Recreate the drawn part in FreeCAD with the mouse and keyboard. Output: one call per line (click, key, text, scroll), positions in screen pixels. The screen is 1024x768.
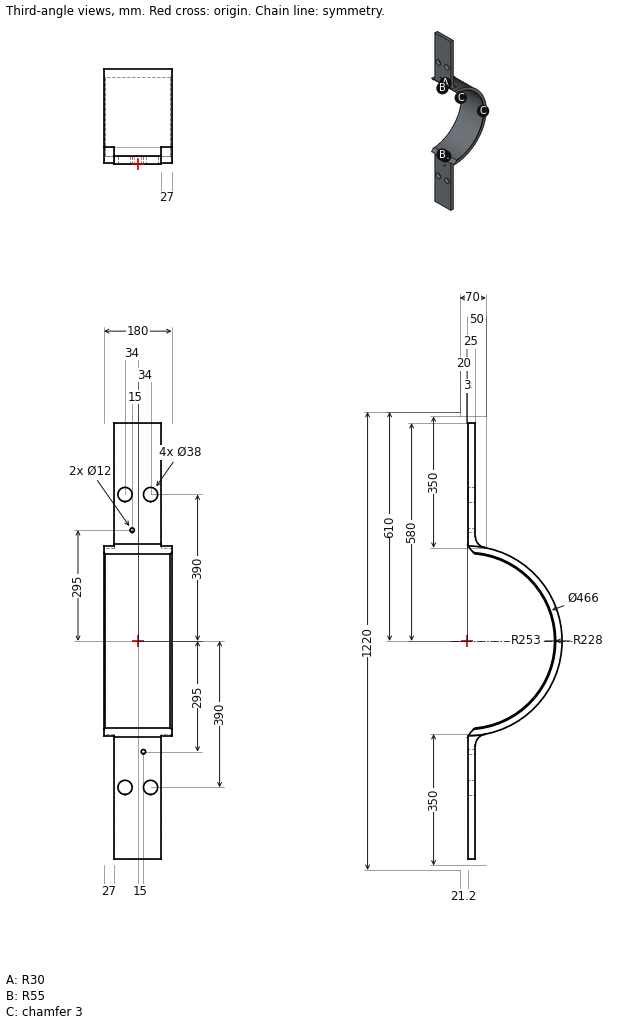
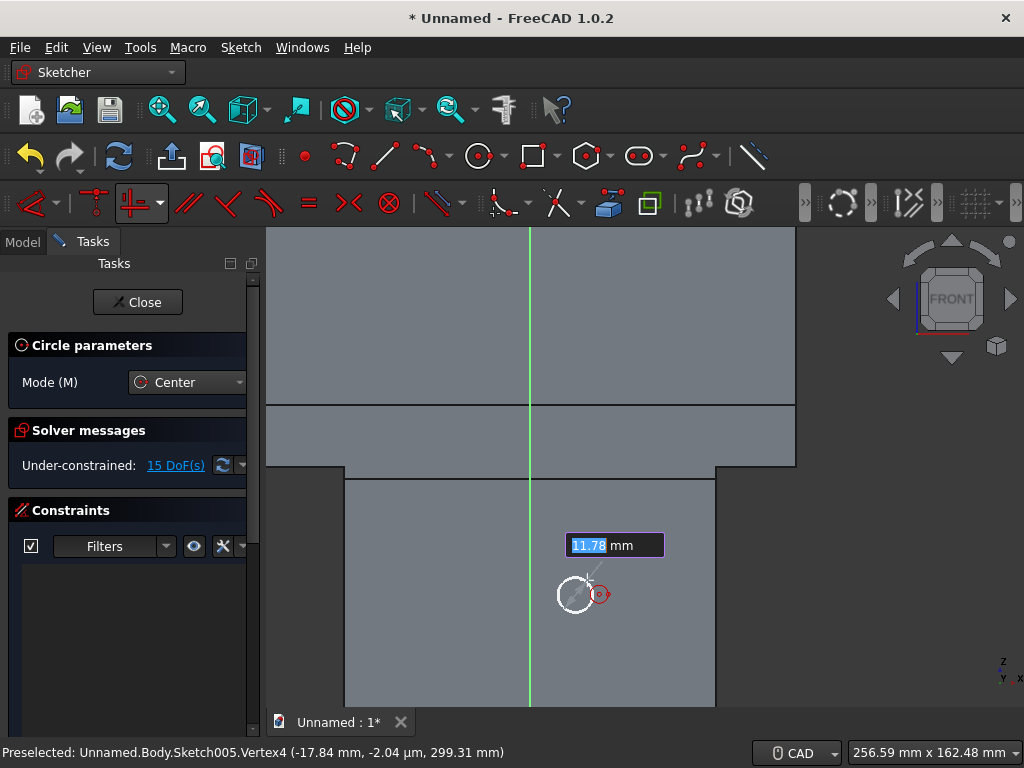
click(587, 579)
key(Escape)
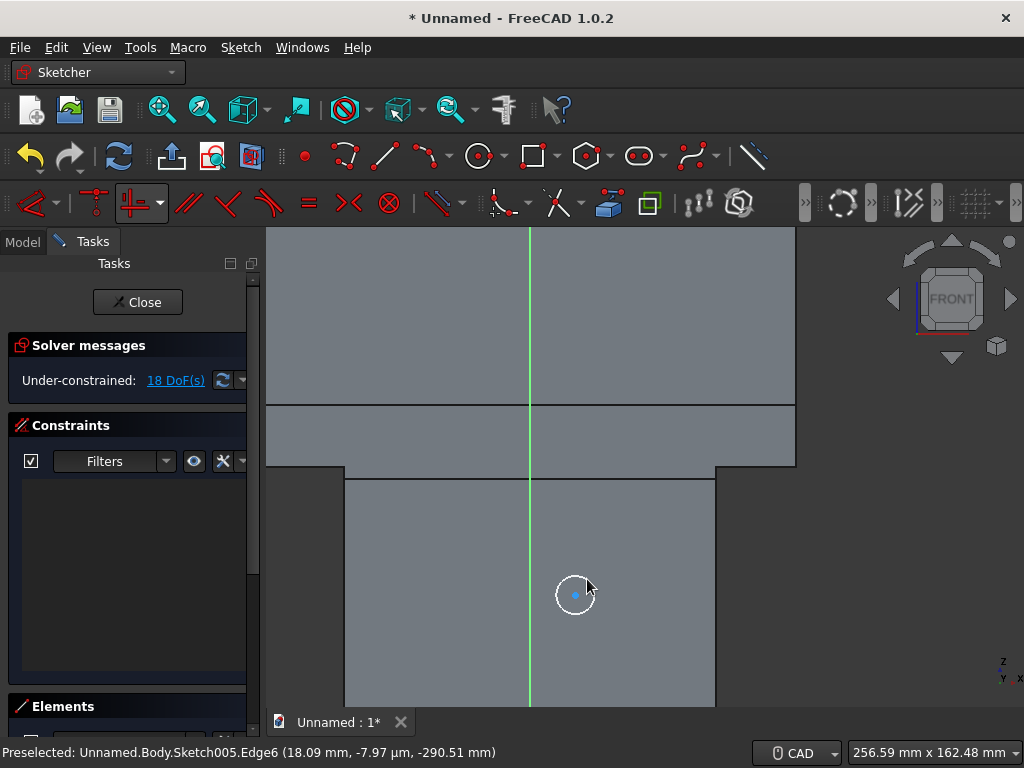
scroll(584, 584, down, 10)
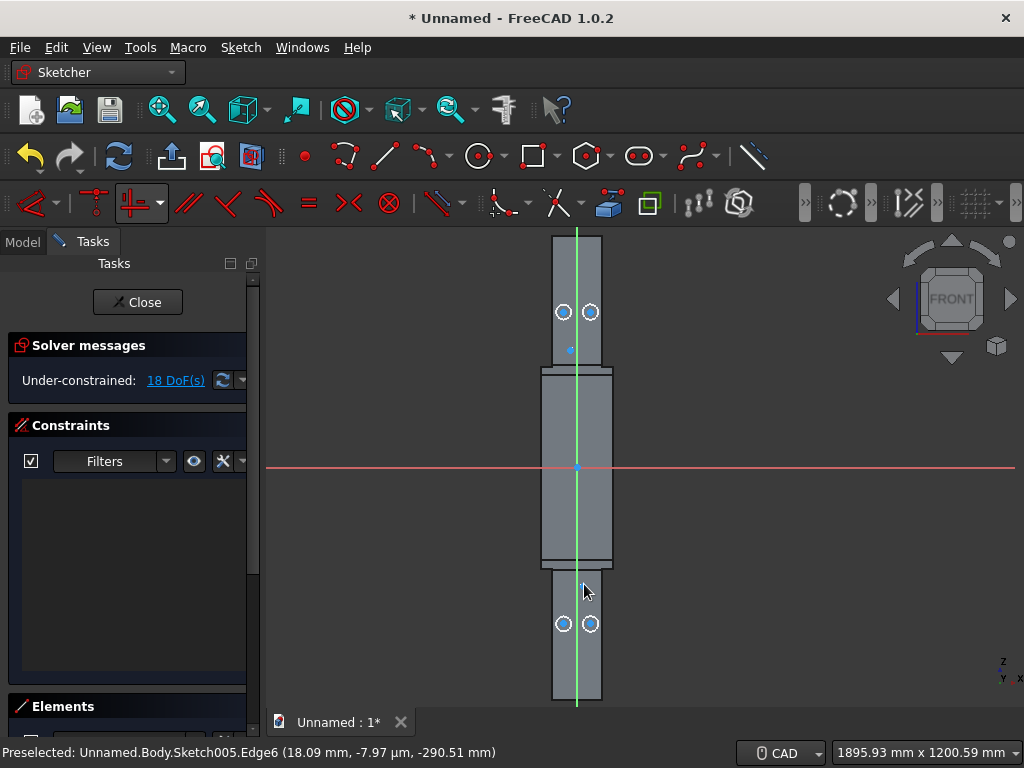
scroll(596, 307, up, 3)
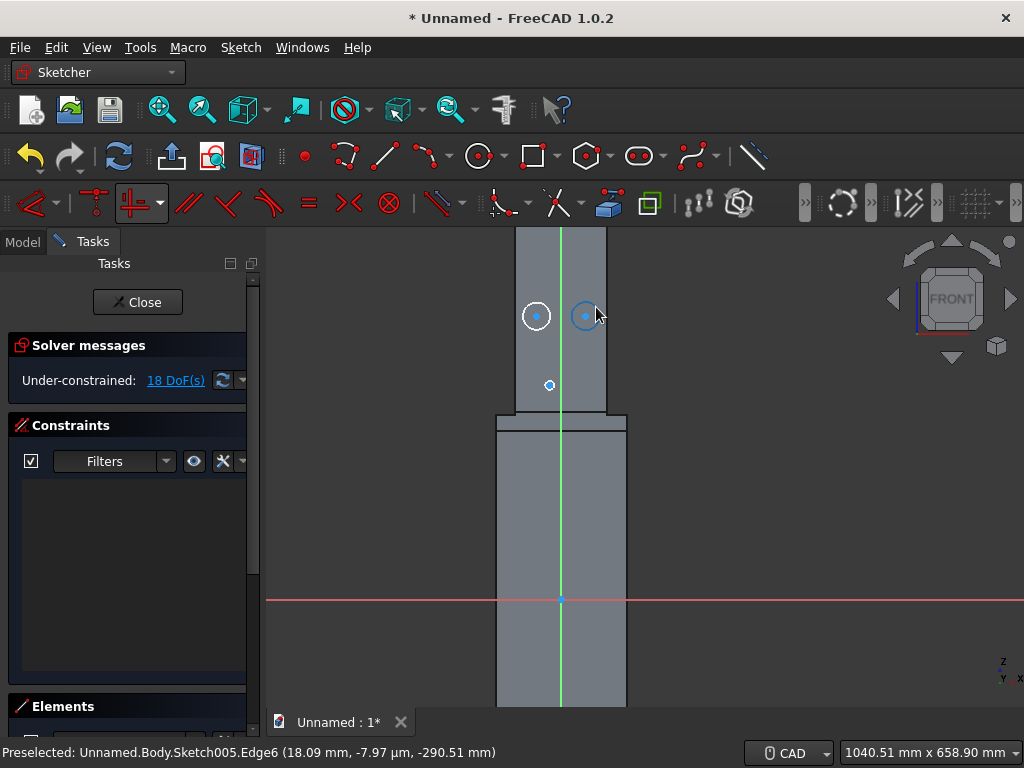
click(596, 306)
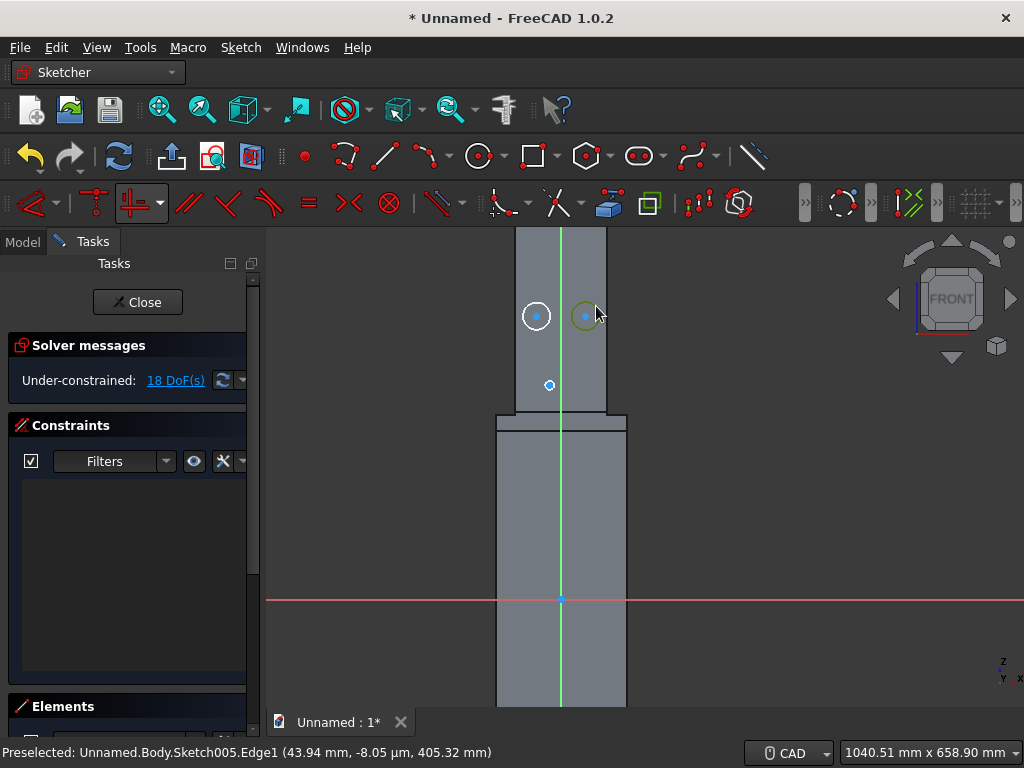
scroll(595, 306, down, 3)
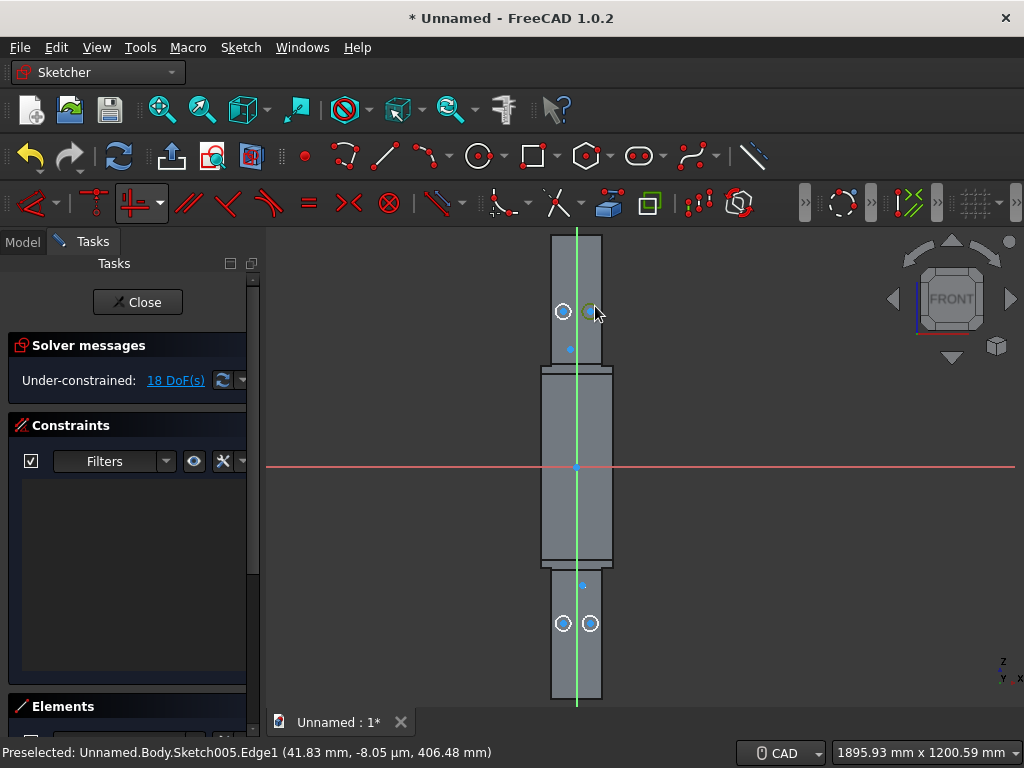
scroll(596, 618, up, 3)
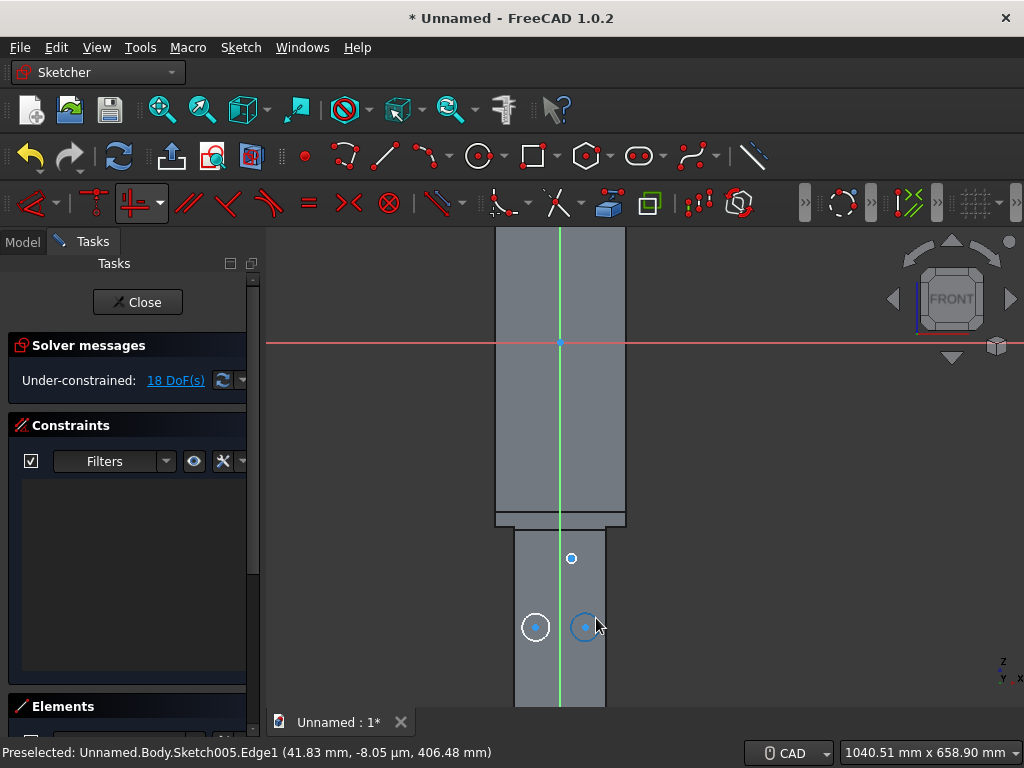
click(595, 617)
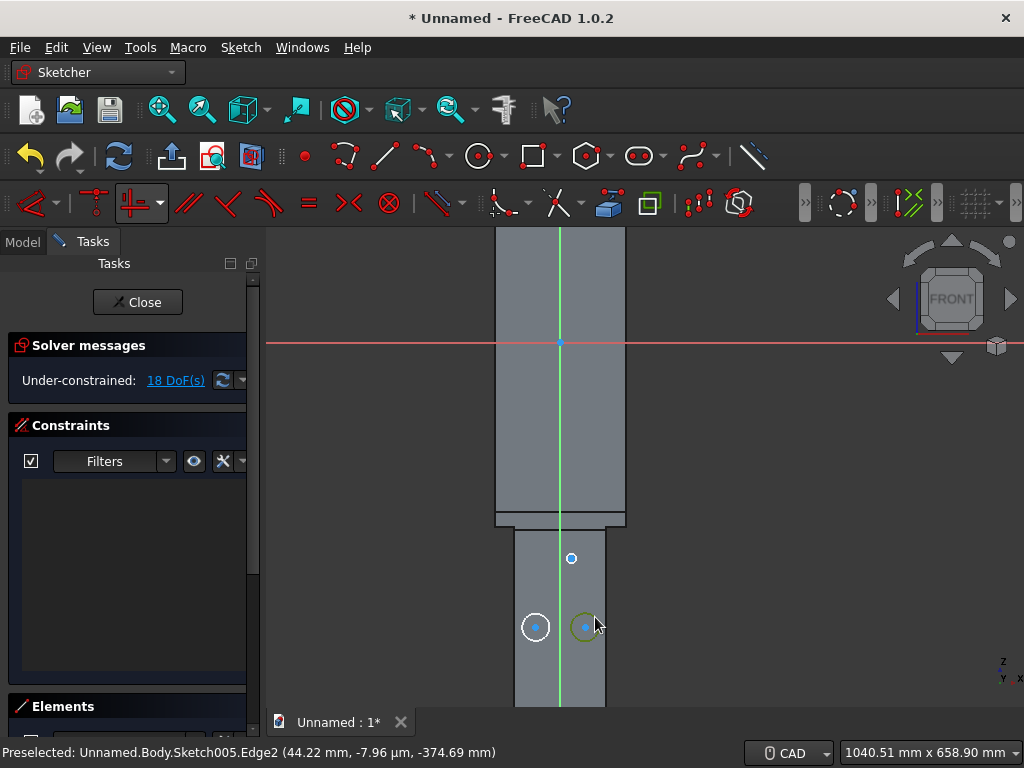
scroll(596, 618, down, 3)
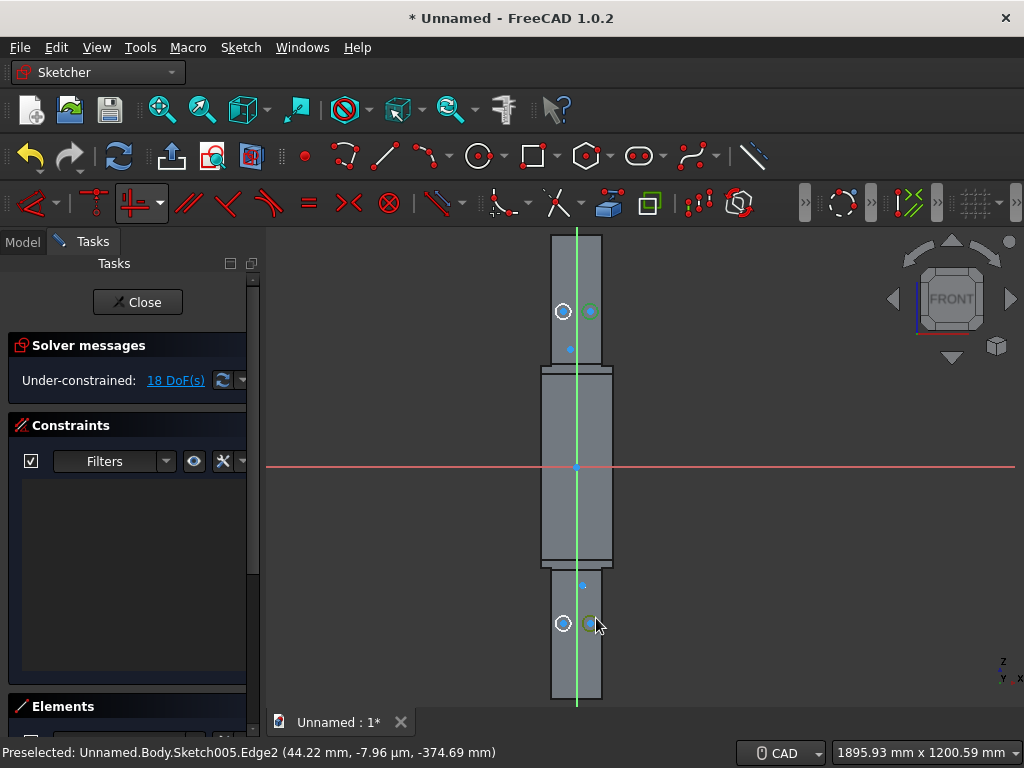
scroll(568, 306, up, 4)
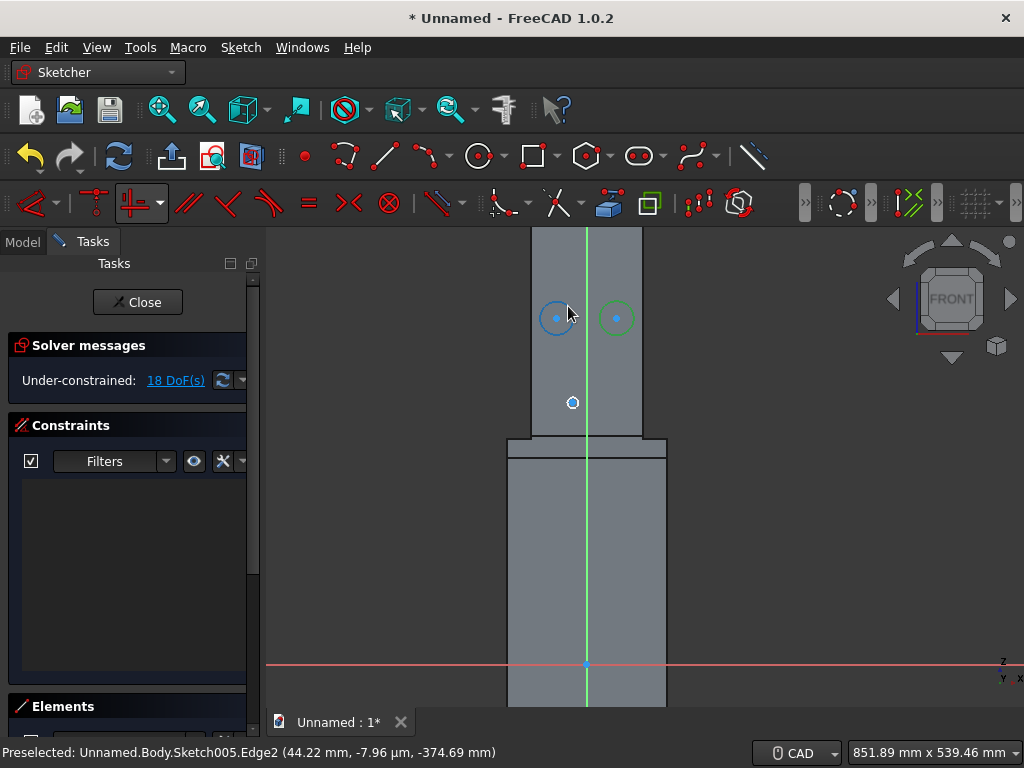
click(568, 307)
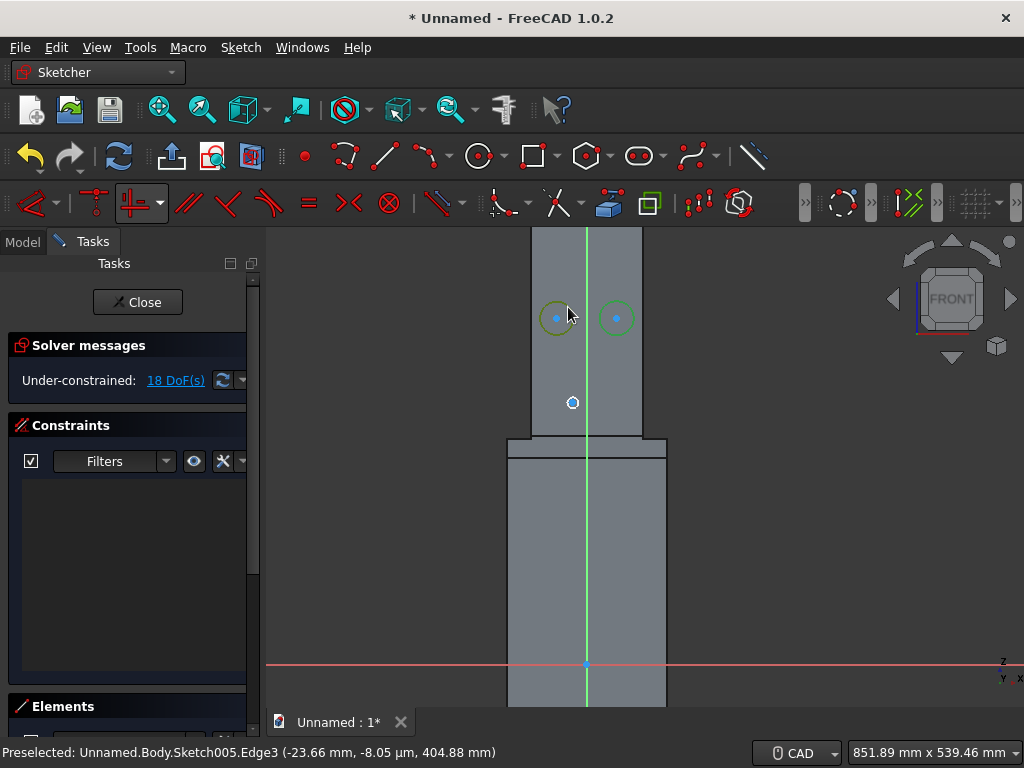
scroll(568, 306, down, 4)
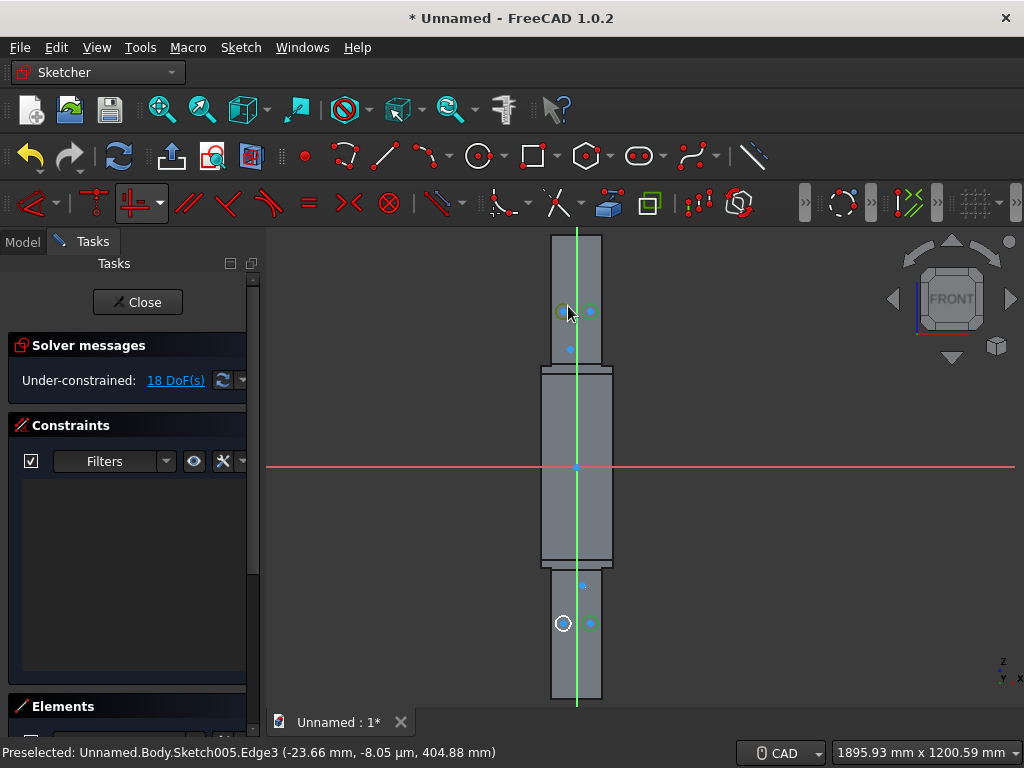
scroll(568, 618, up, 4)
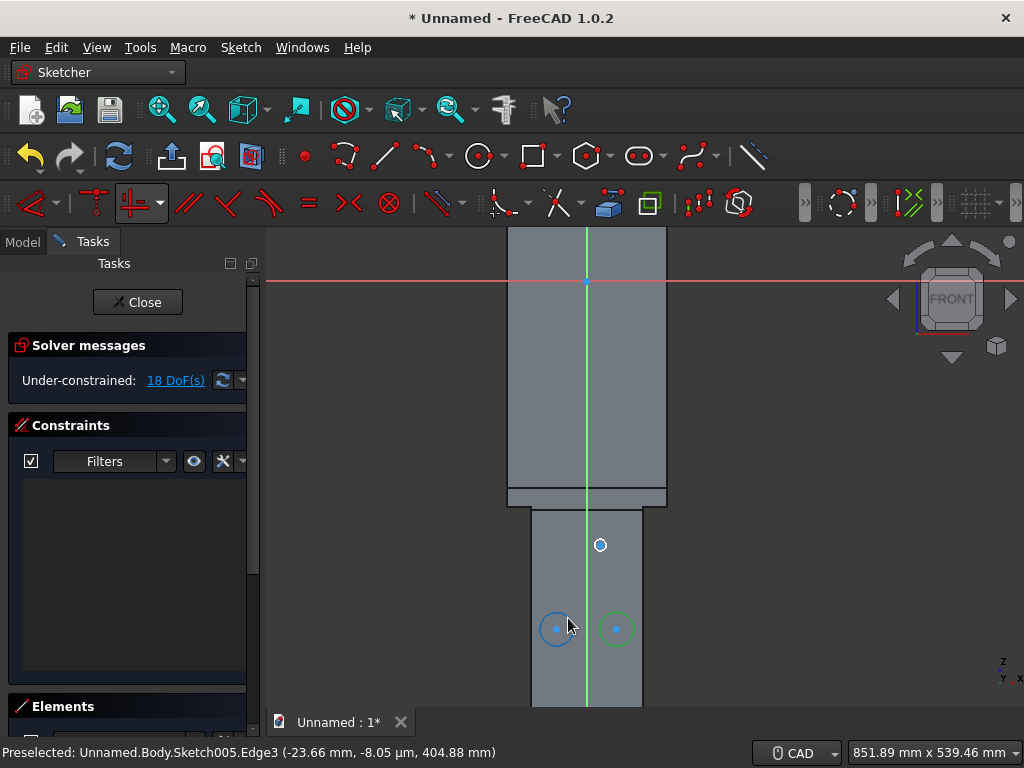
click(568, 617)